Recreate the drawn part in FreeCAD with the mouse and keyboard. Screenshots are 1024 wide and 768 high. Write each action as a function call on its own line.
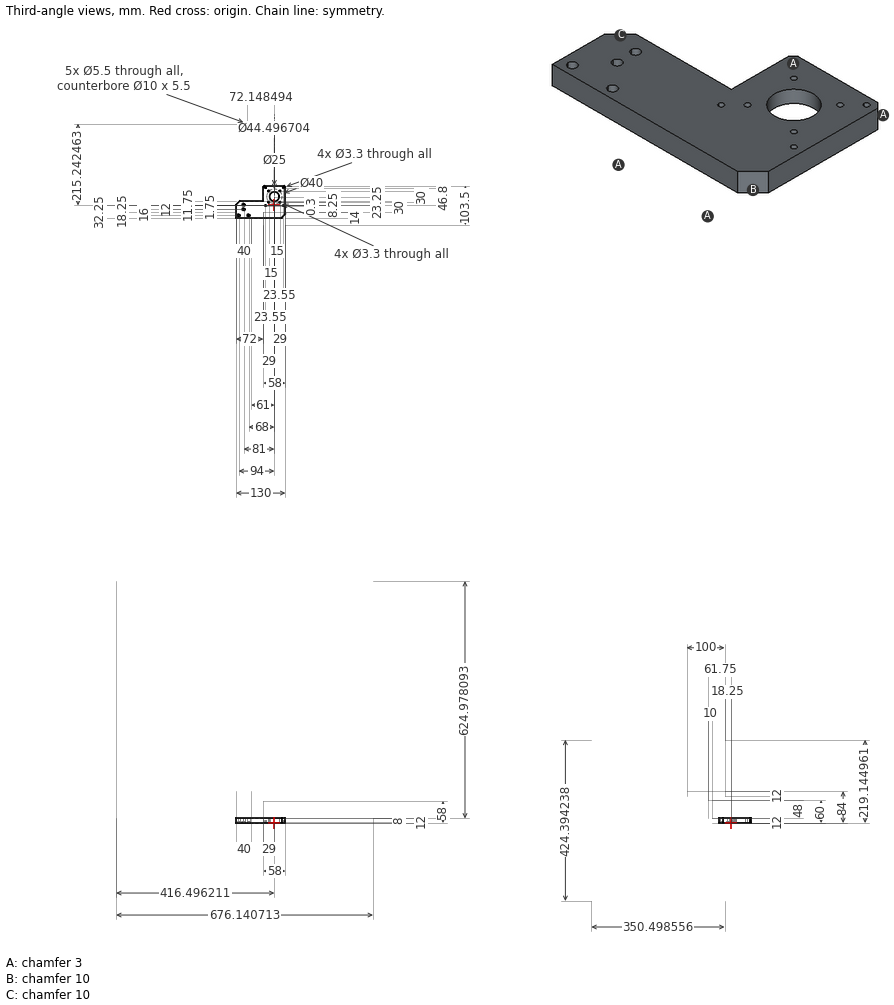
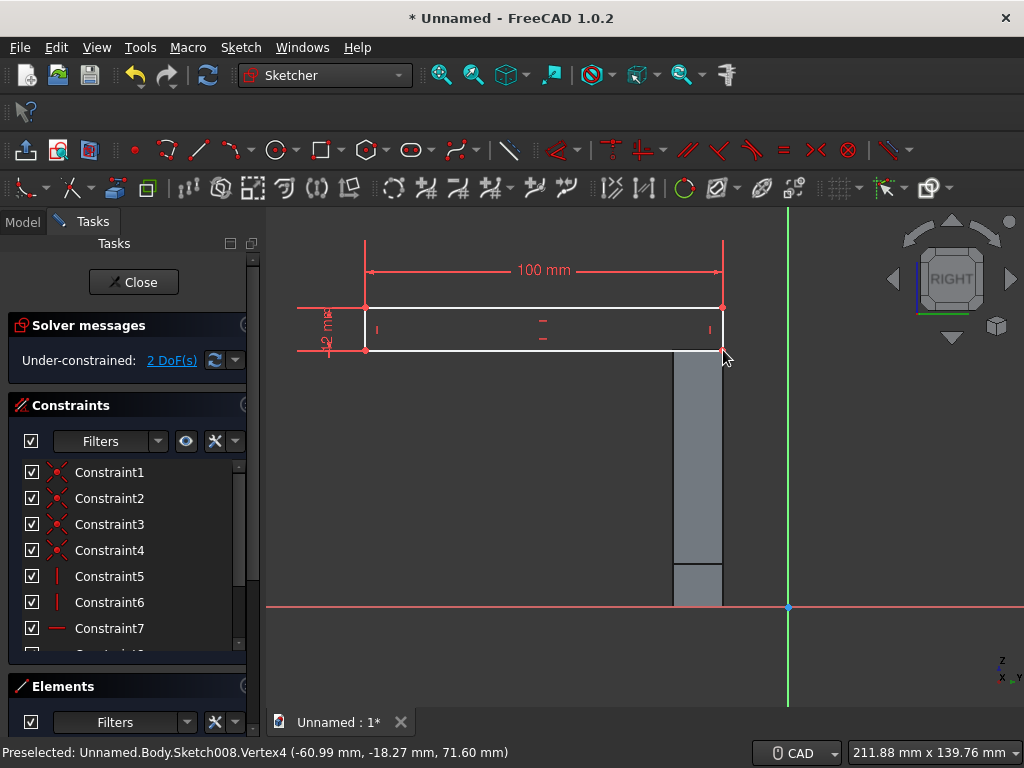
click(556, 150)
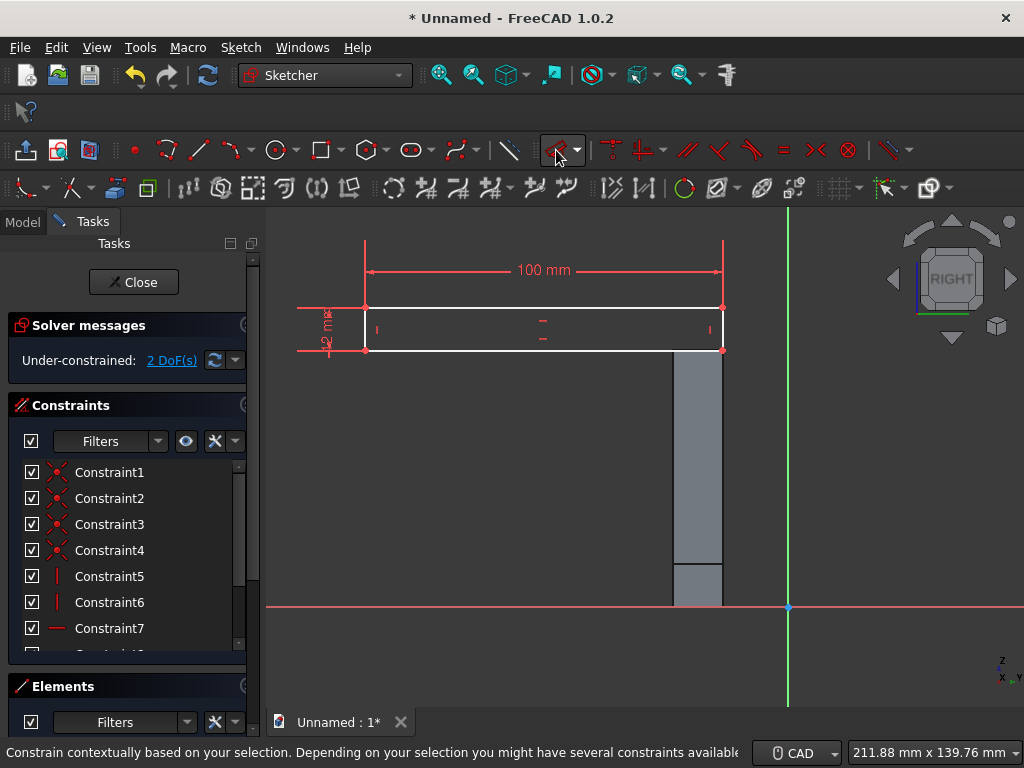
click(365, 308)
click(331, 458)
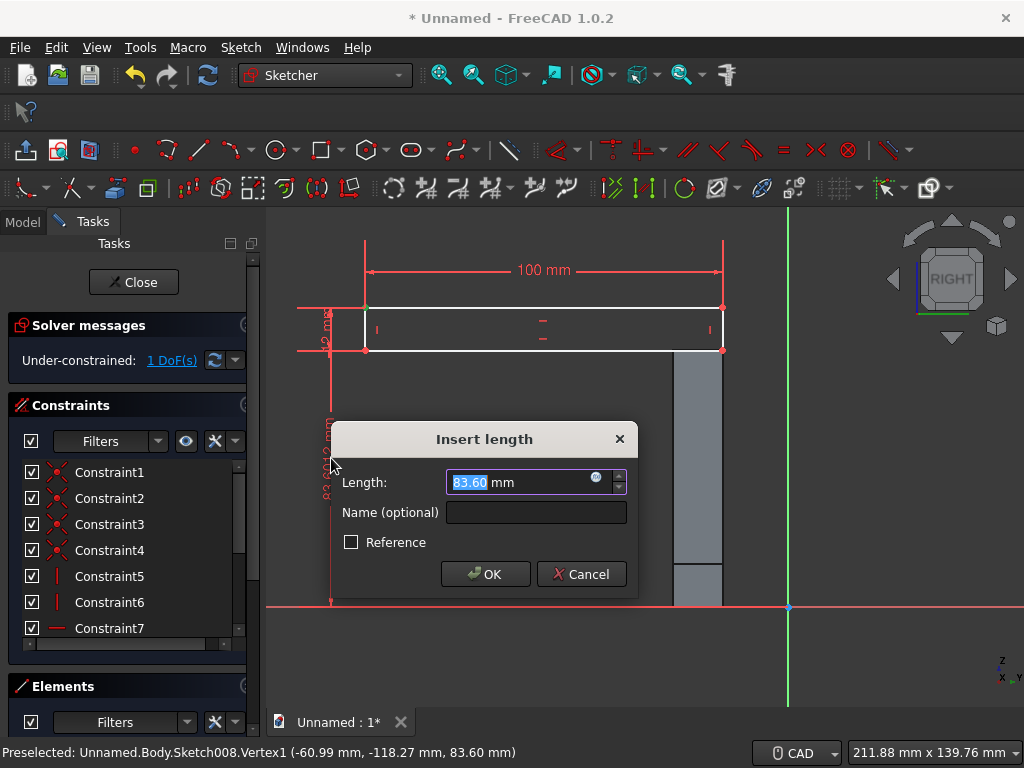
text(84)
key(Return)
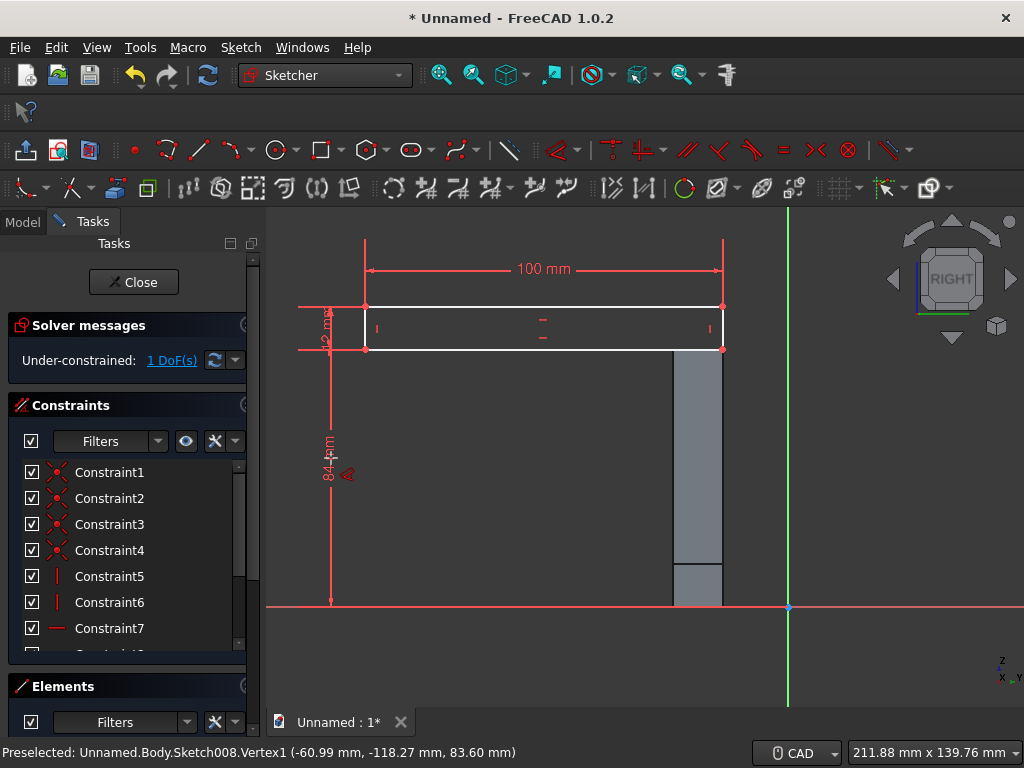
click(723, 350)
click(755, 641)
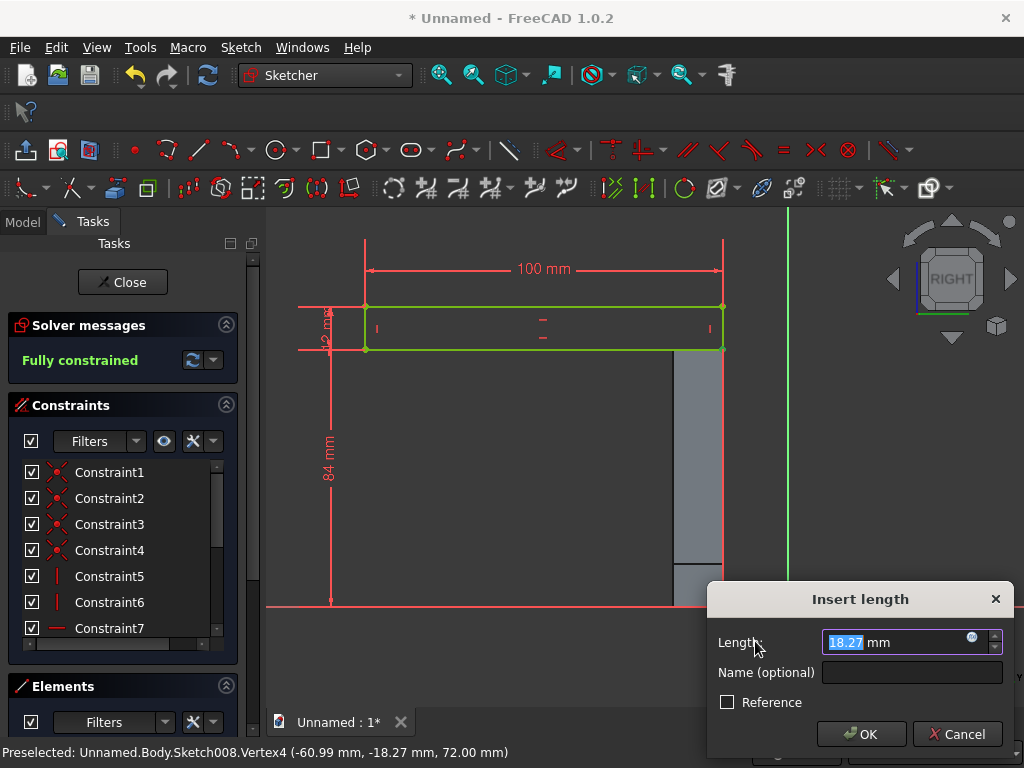
text(18.25)
key(Return)
key(Escape)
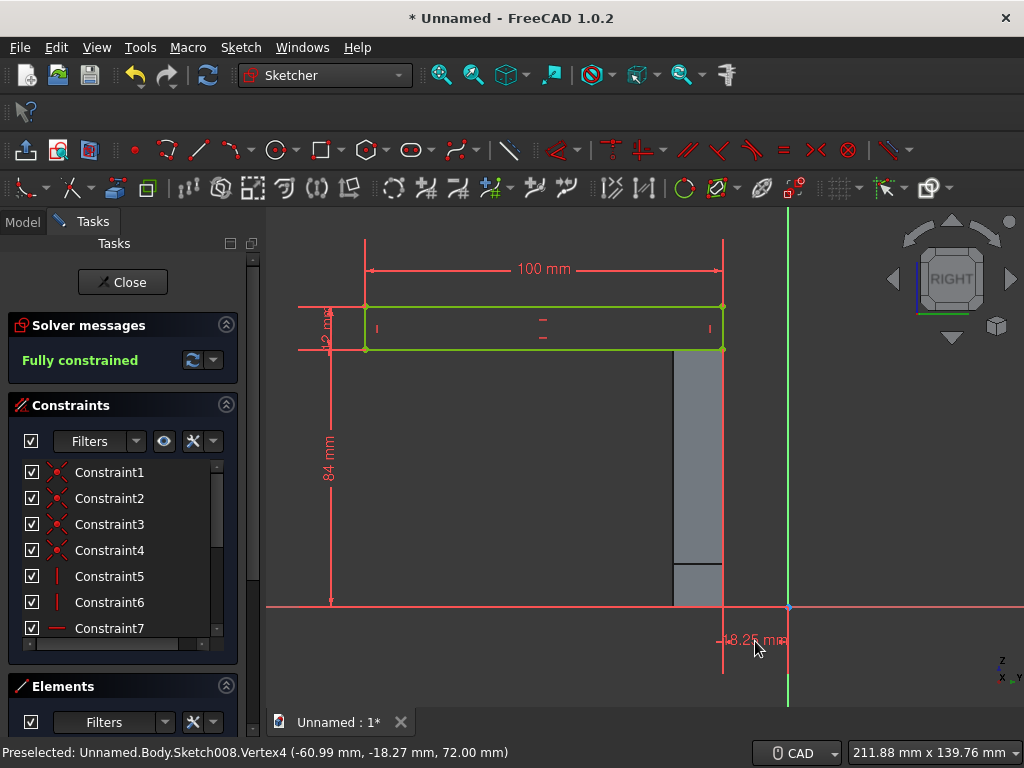
click(123, 282)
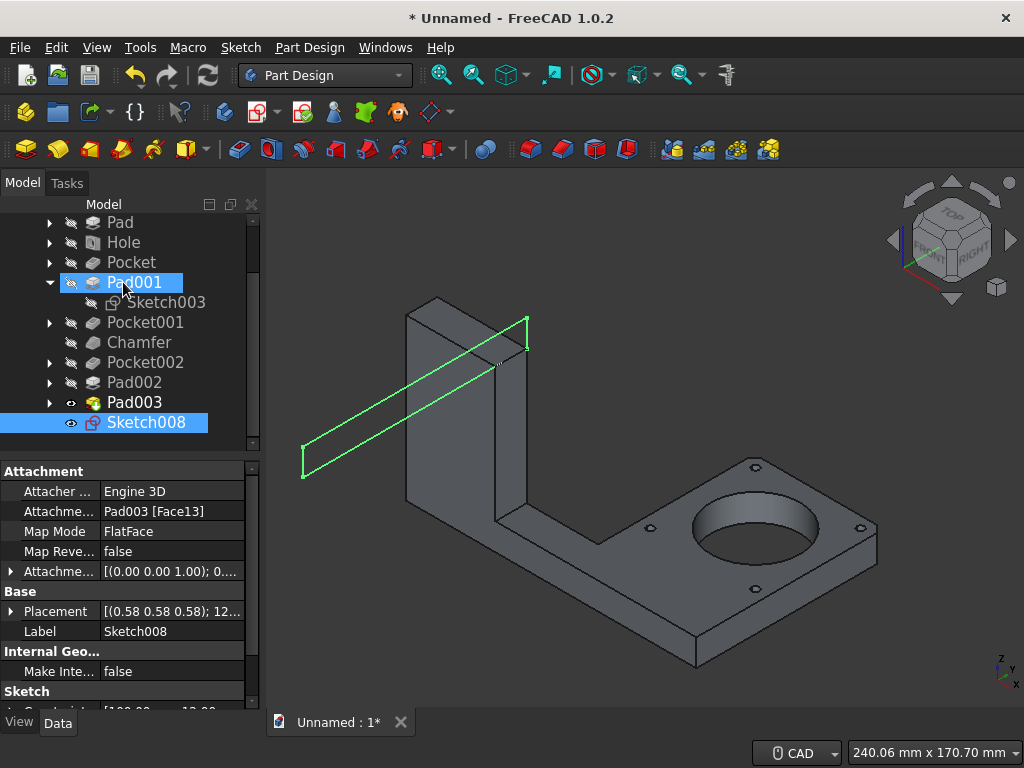
click(26, 150)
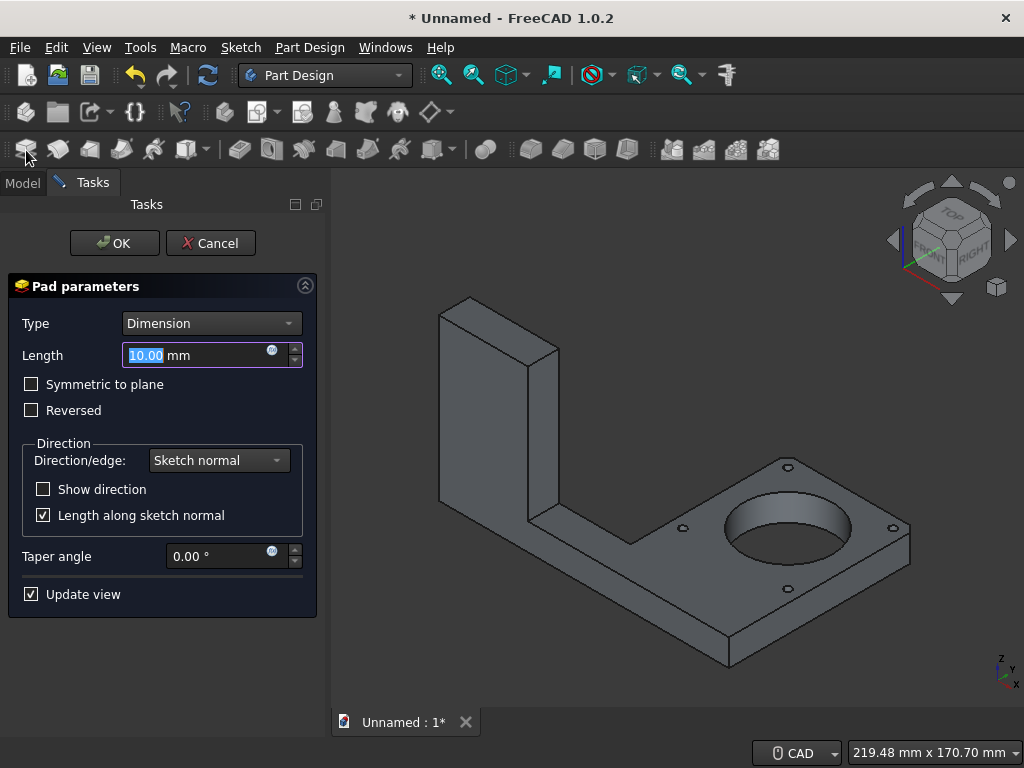
text(40)
key(Tab)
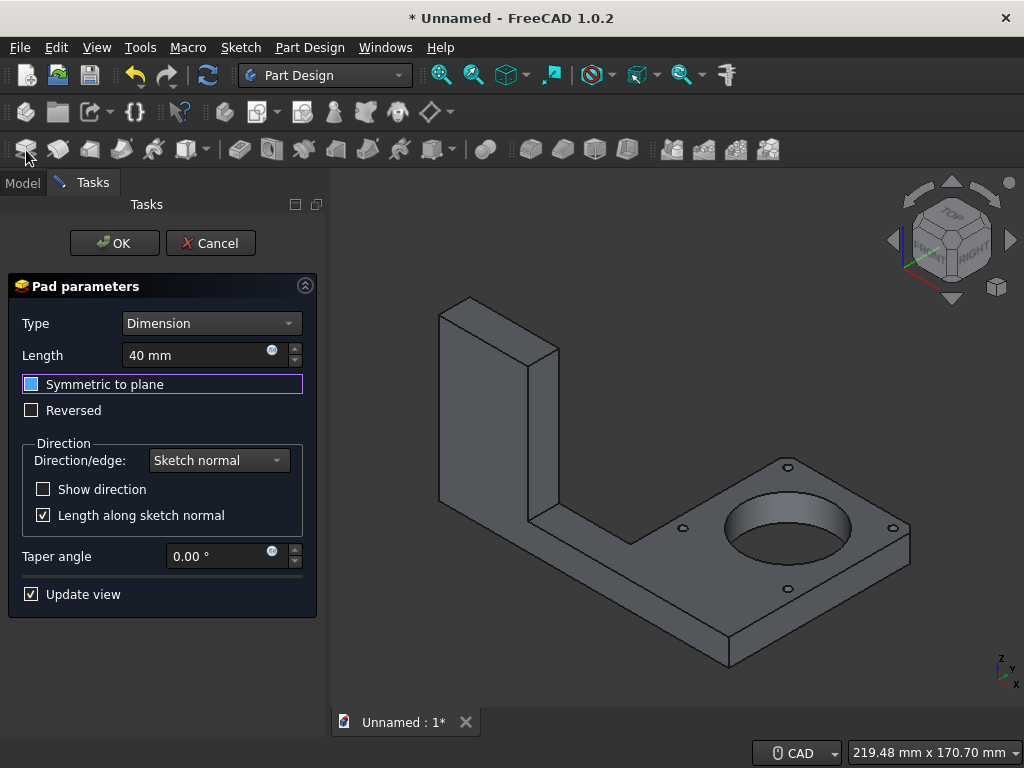
click(30, 410)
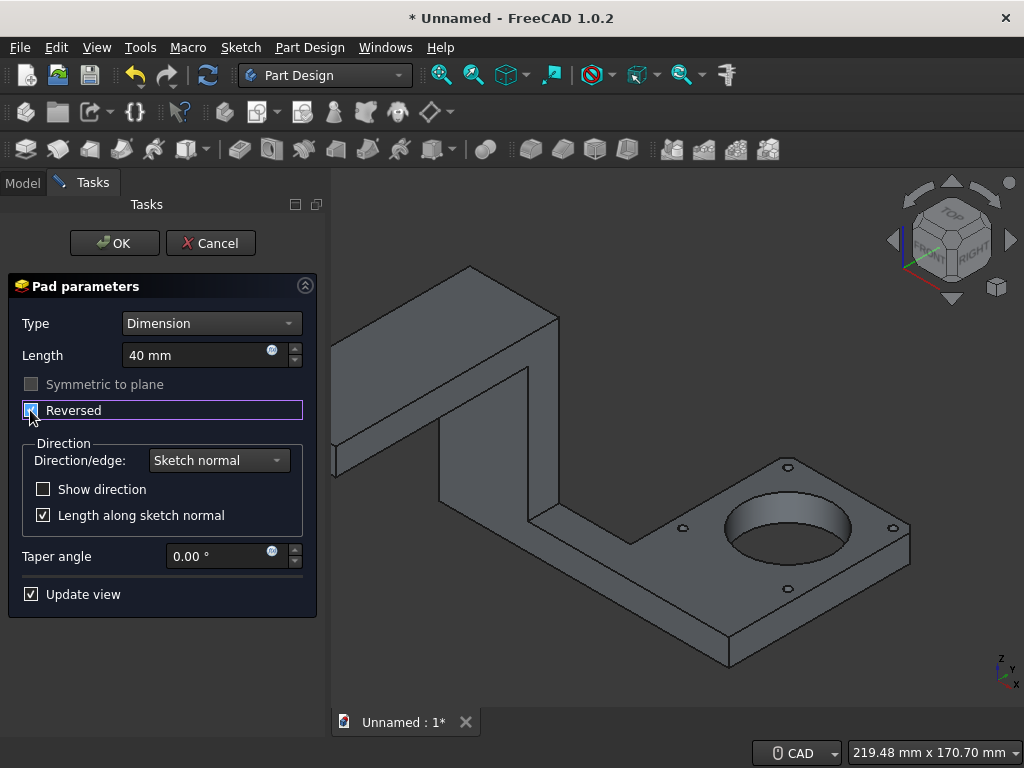
click(115, 243)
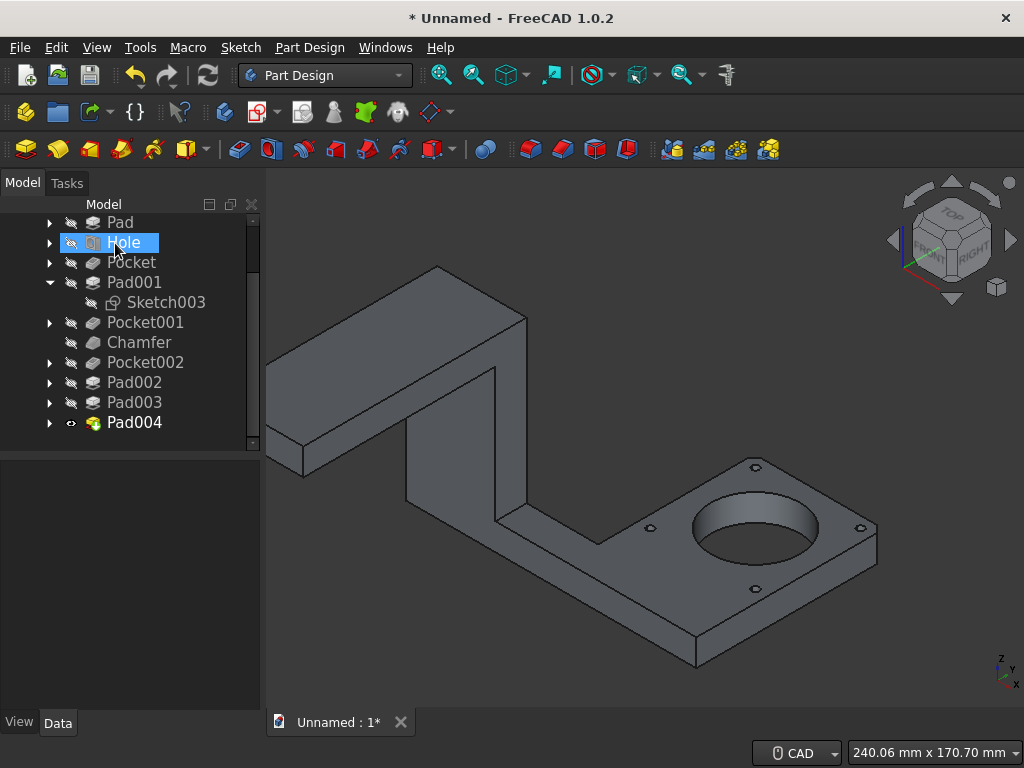
click(442, 76)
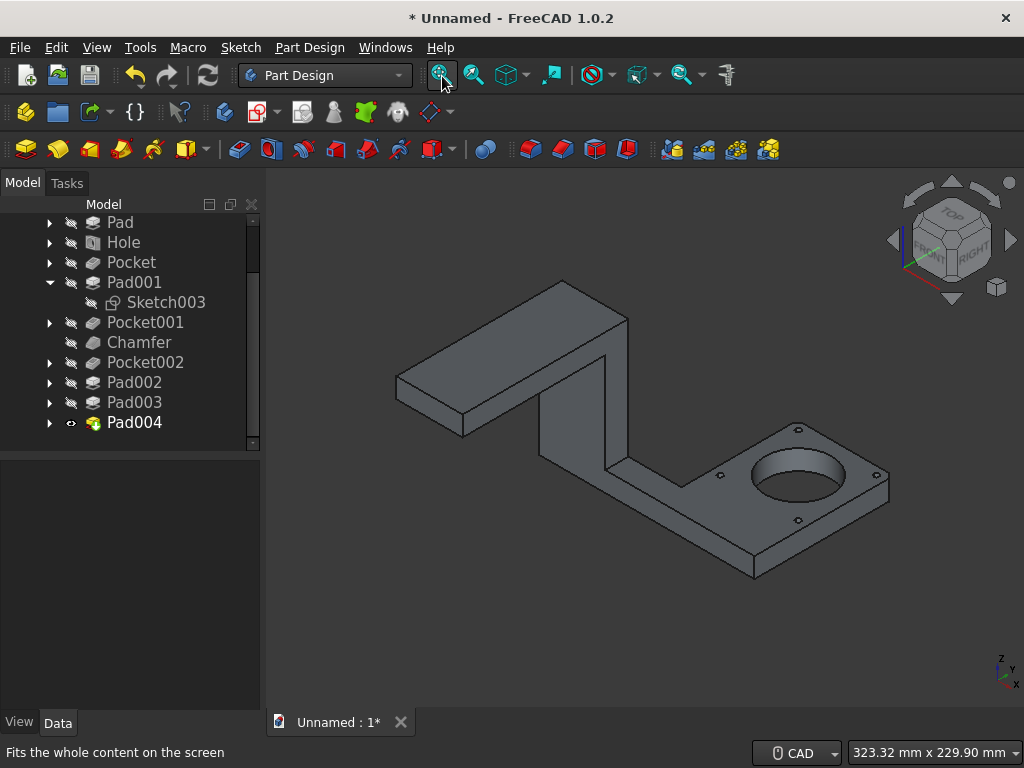
click(752, 519)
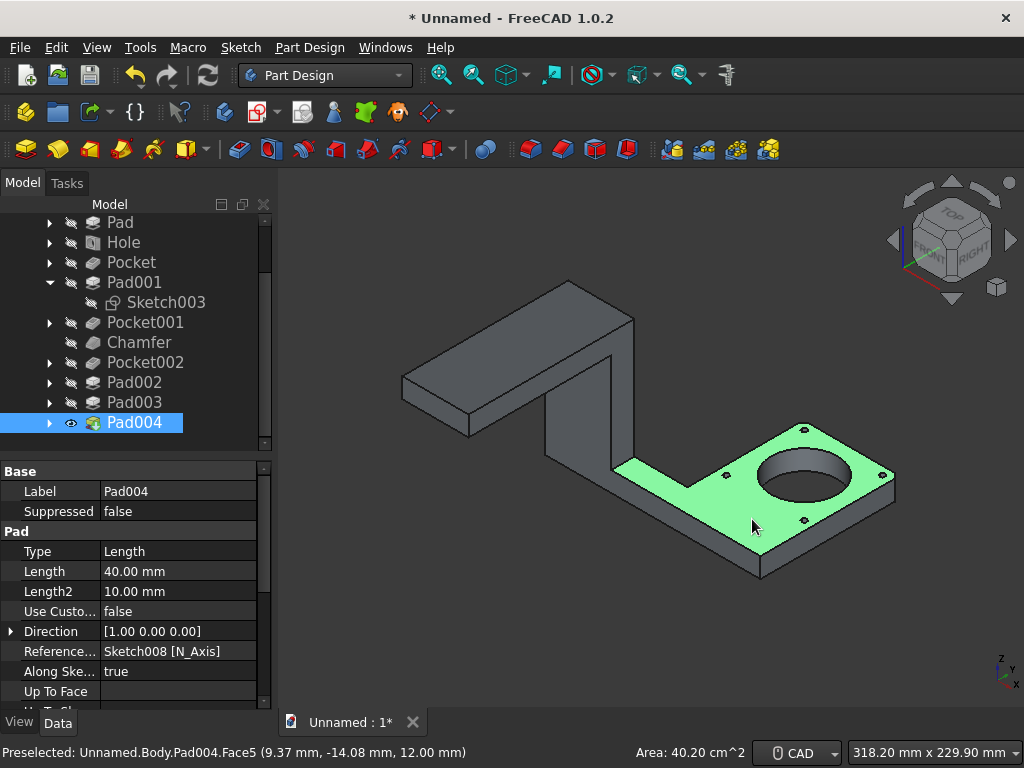
click(258, 112)